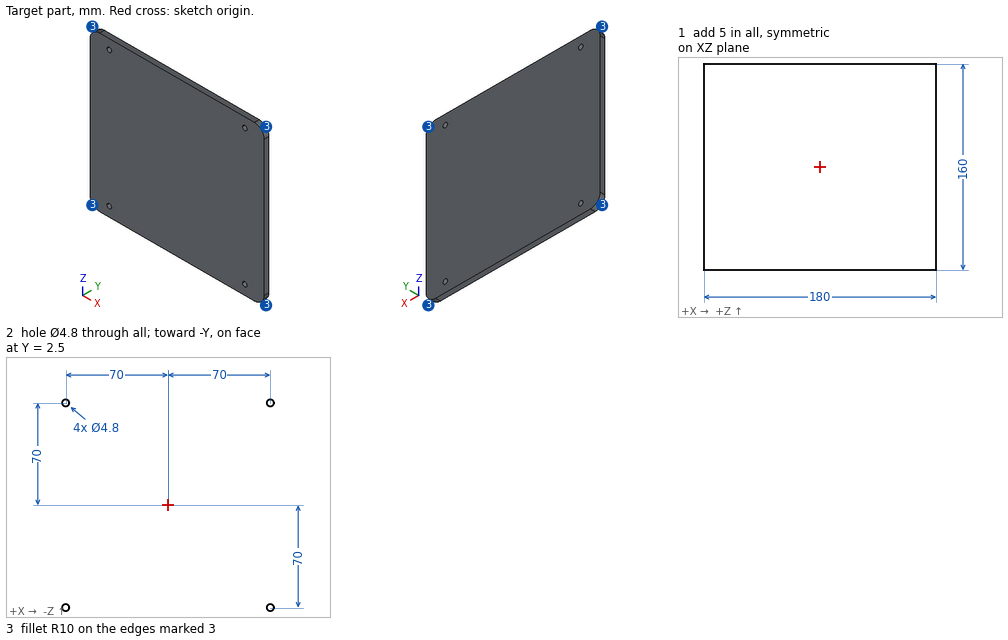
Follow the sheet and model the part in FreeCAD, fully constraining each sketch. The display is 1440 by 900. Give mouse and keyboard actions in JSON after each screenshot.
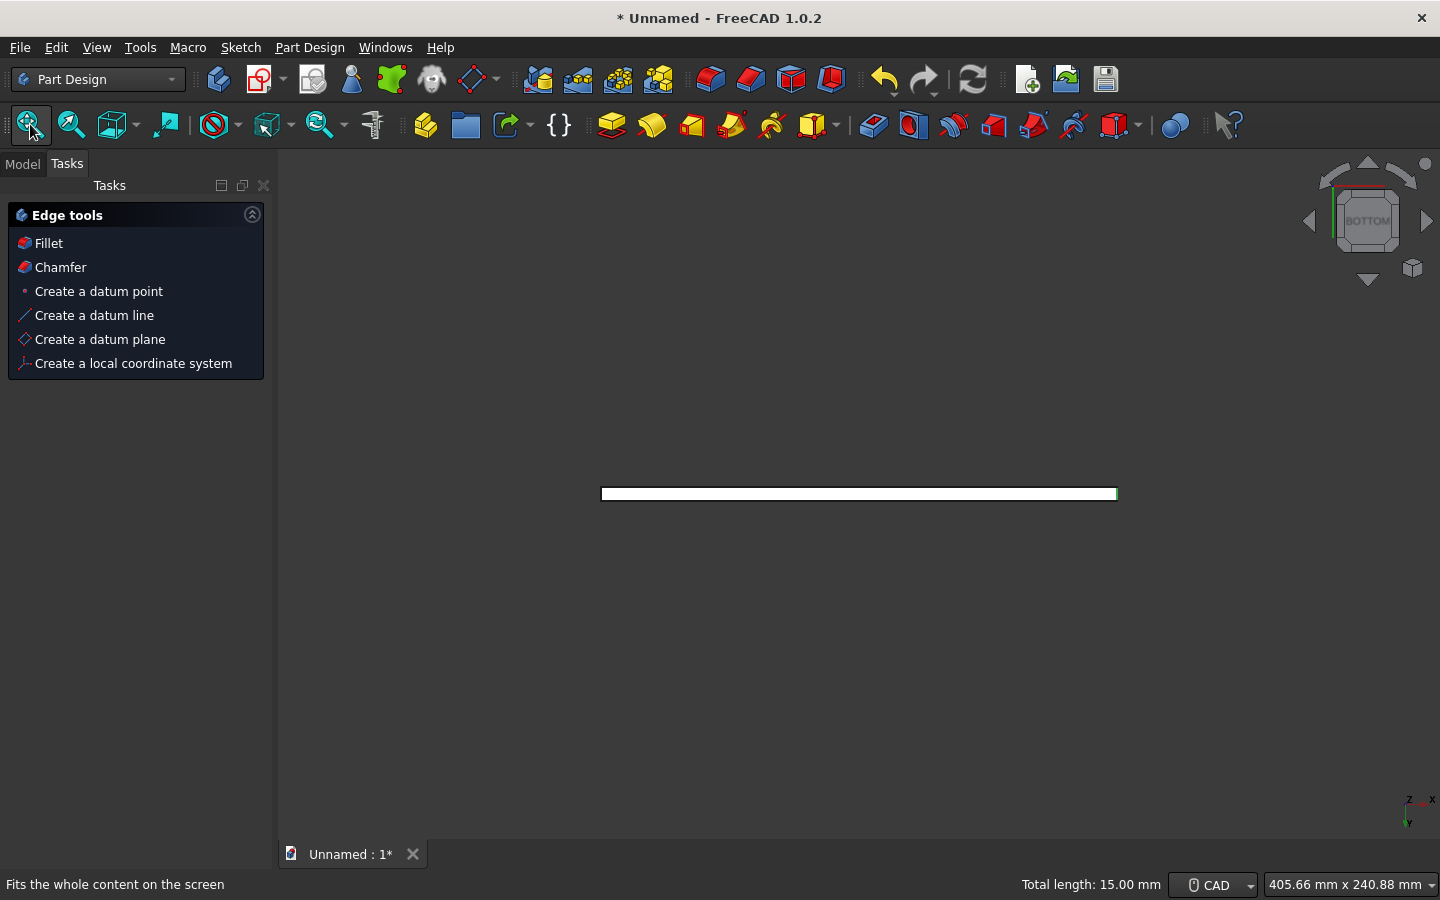
{"action": "left_click", "coordinate": [601, 493], "text": "ctrl"}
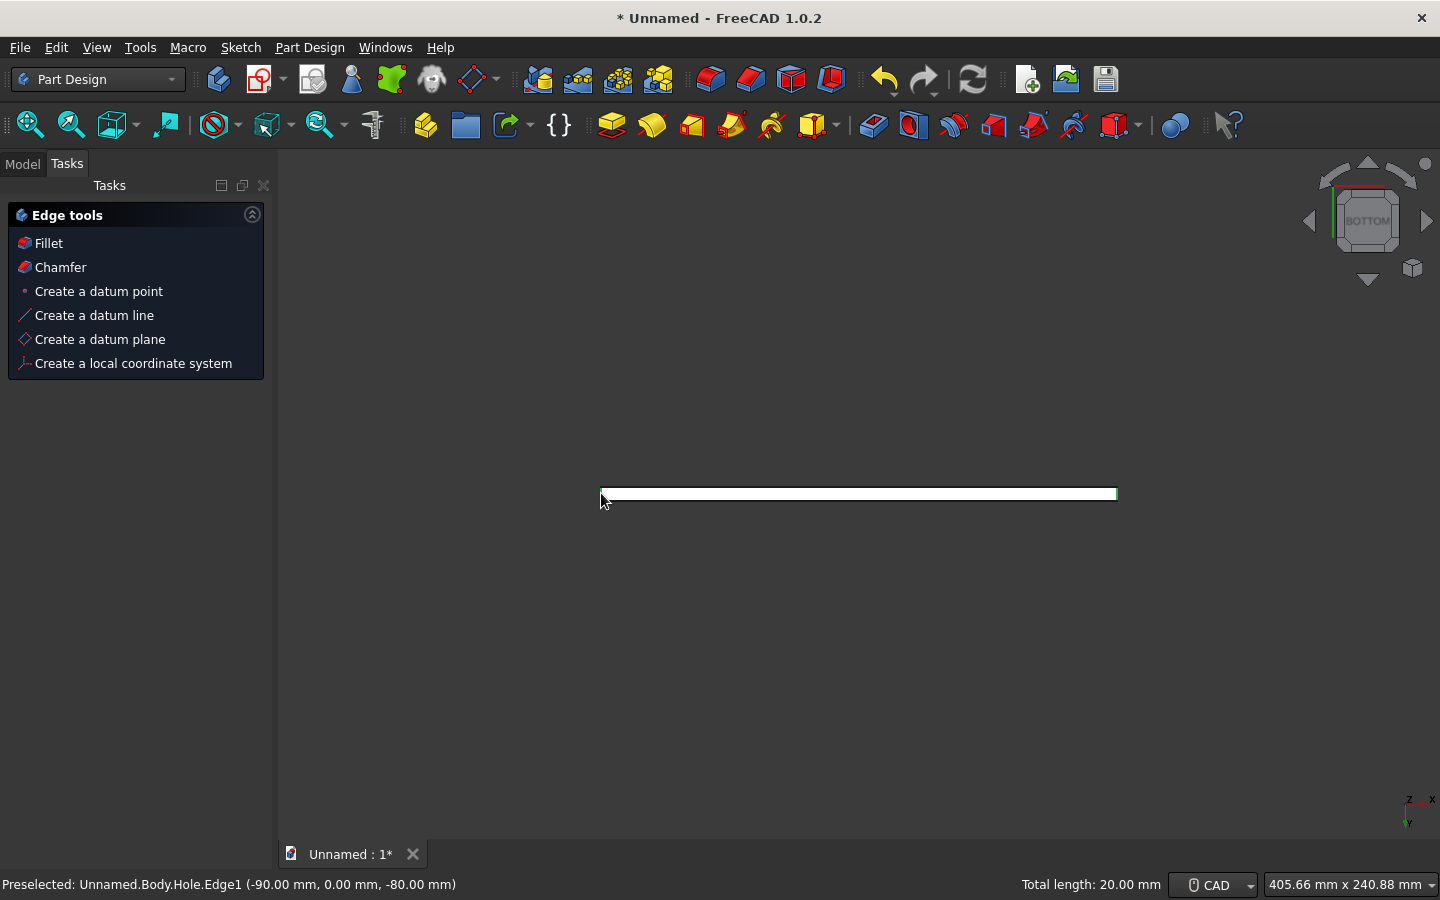
{"action": "left_click", "coordinate": [712, 80]}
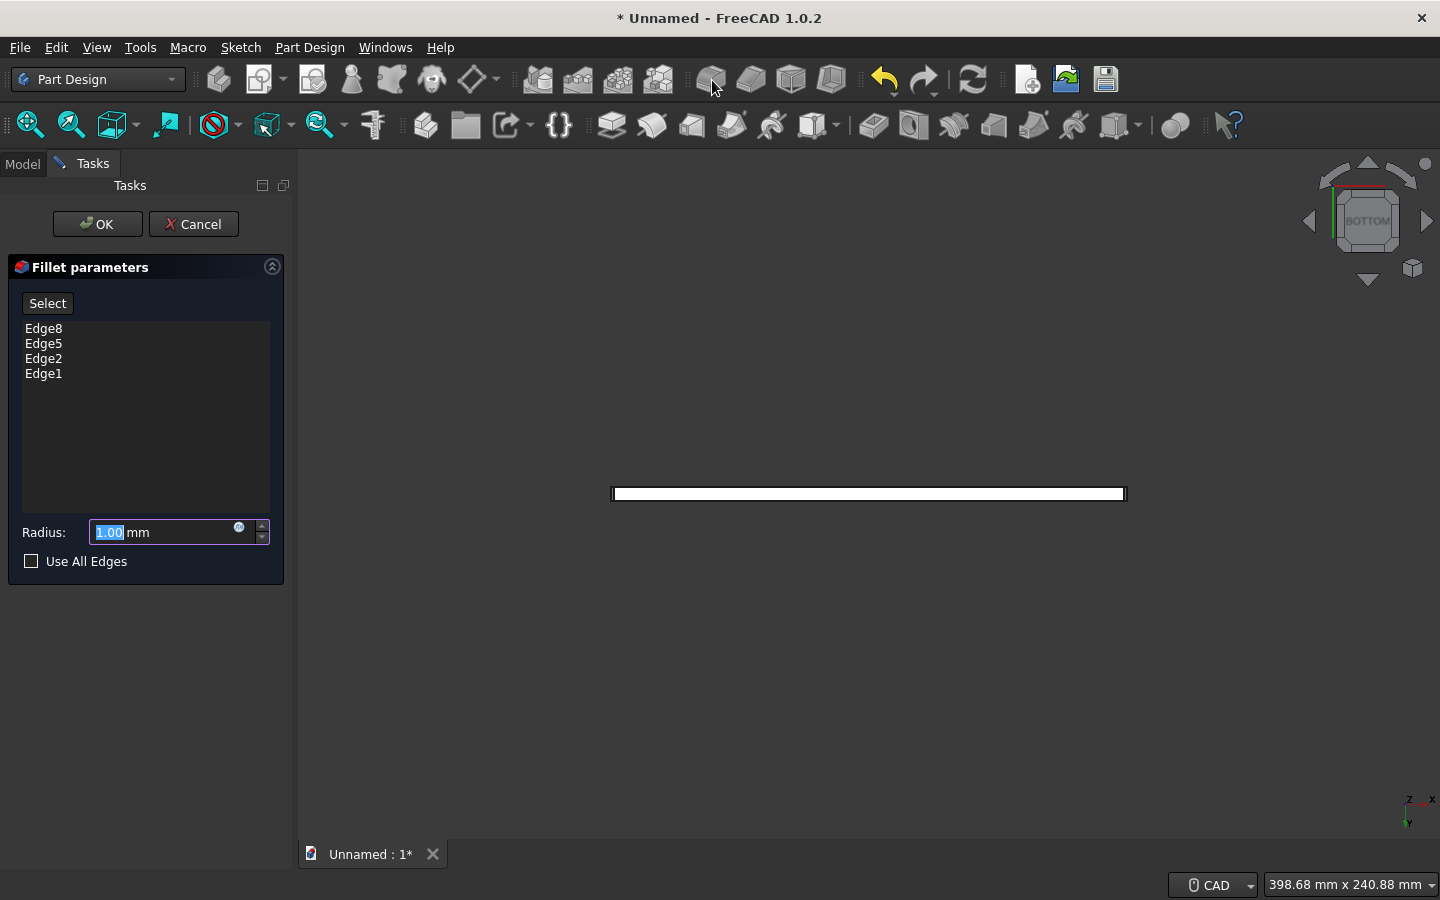
{"action": "type", "text": "10"}
{"action": "key", "text": "Tab"}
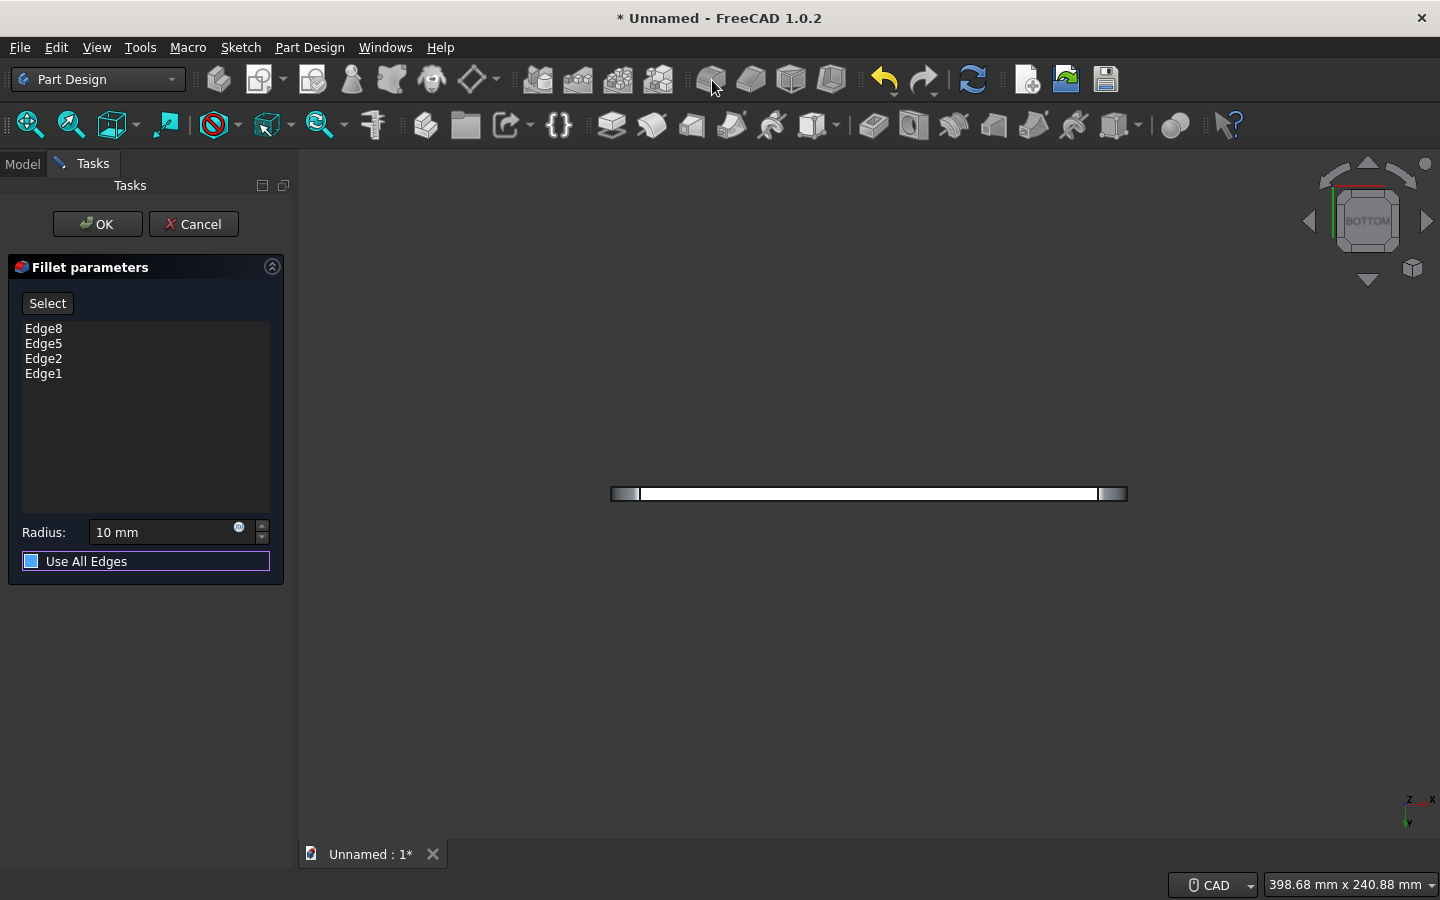
{"action": "left_click", "coordinate": [98, 224]}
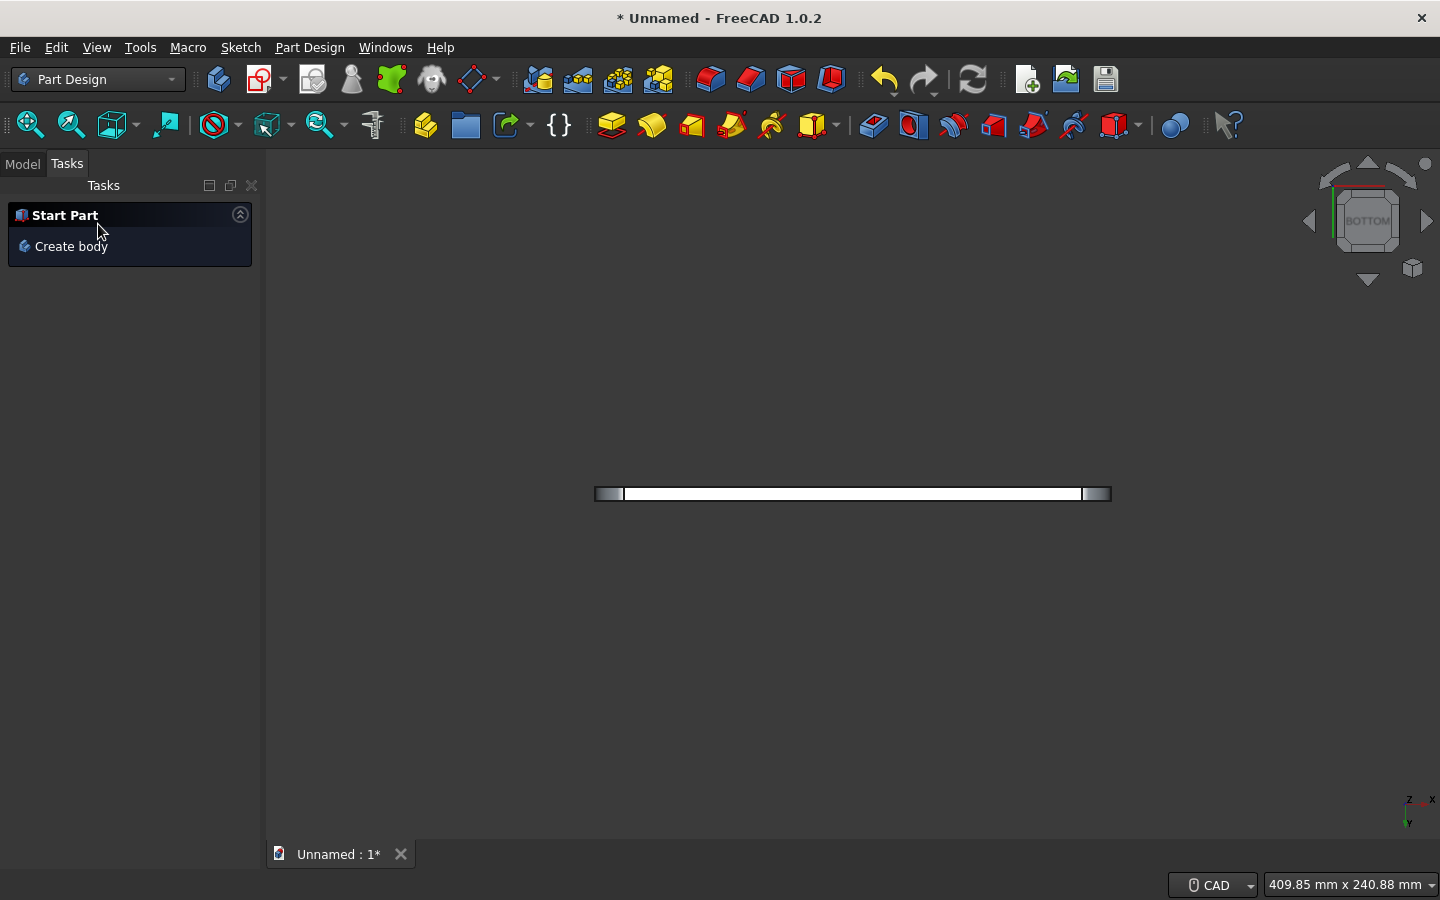
{"action": "key", "text": "0"}